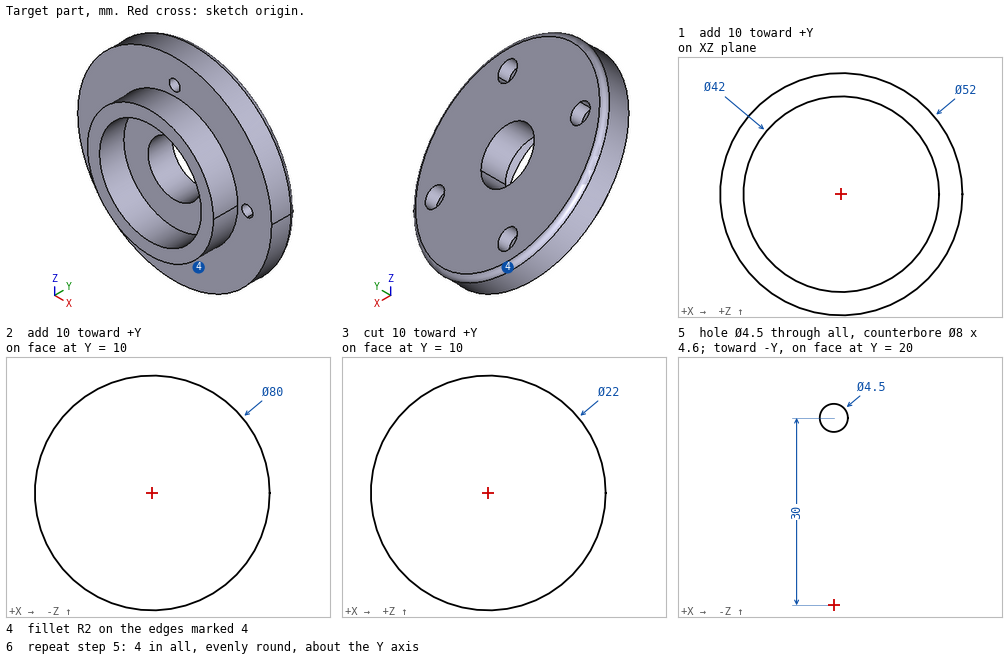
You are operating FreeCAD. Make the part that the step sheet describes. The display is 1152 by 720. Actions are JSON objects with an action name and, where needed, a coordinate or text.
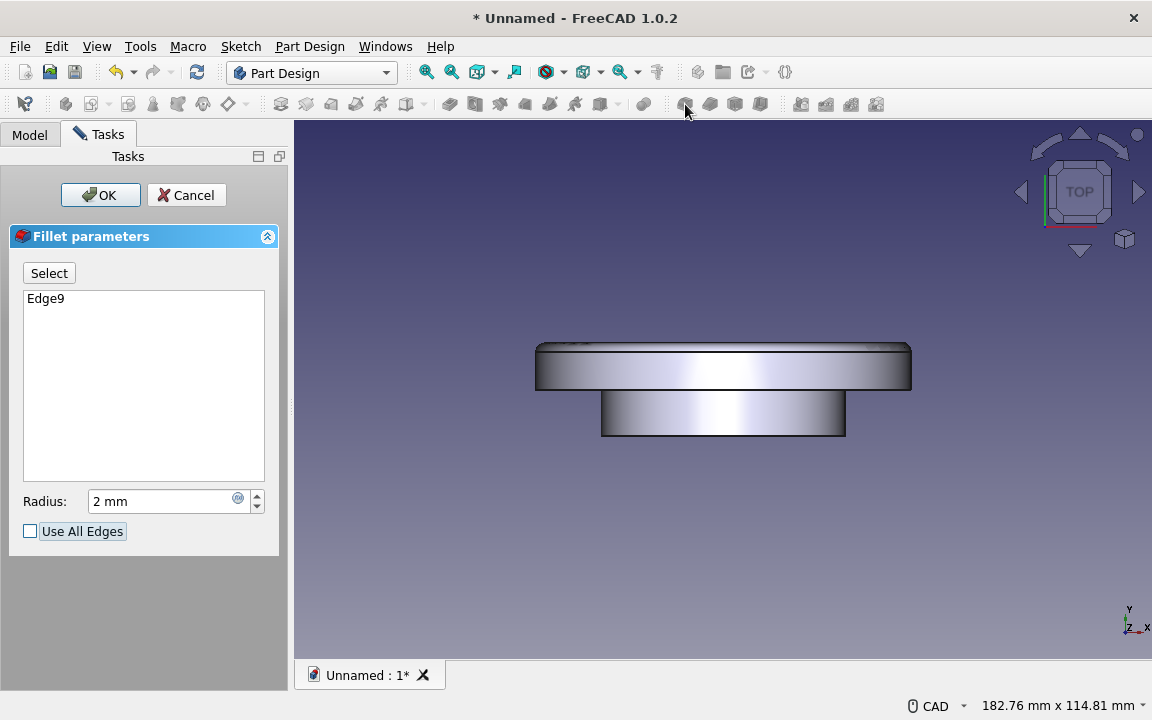
{"action": "left_click", "coordinate": [101, 195]}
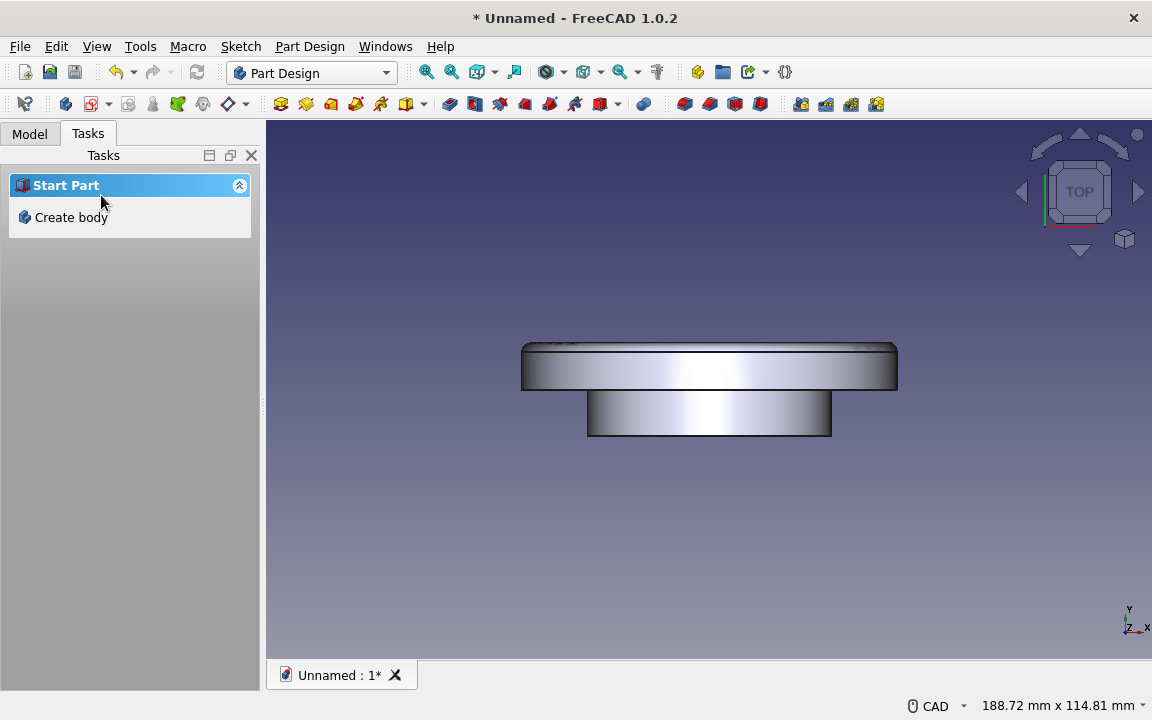
{"action": "key", "text": "v f"}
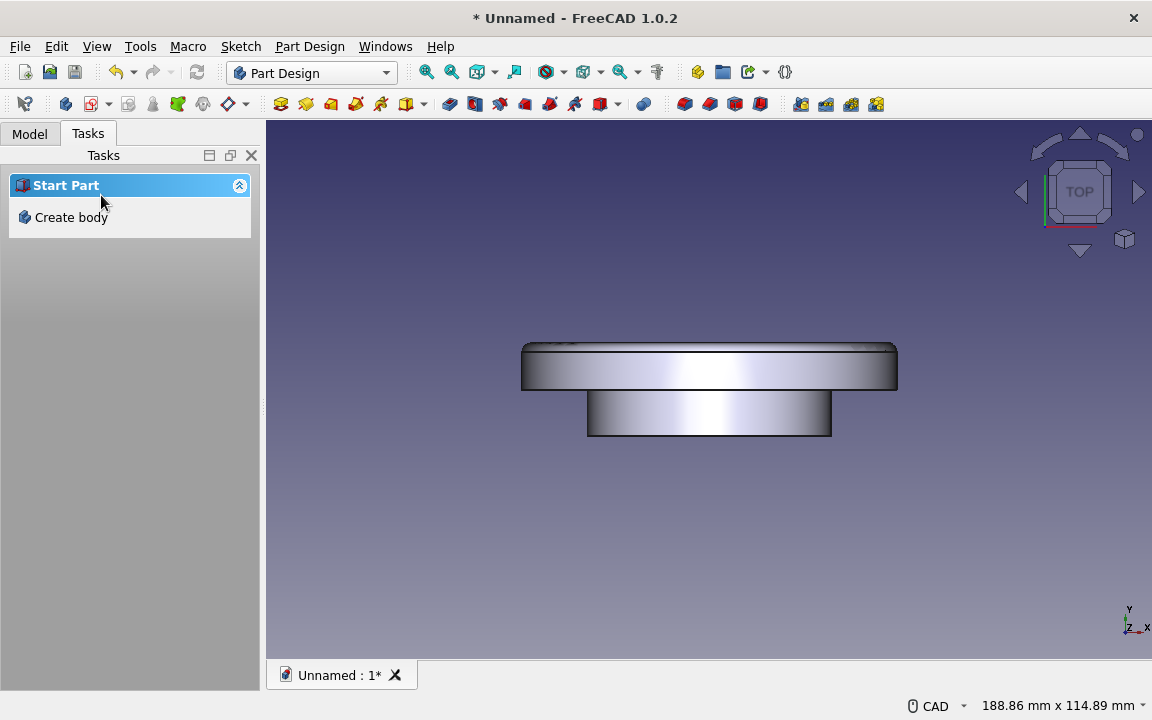
{"action": "key", "text": "4"}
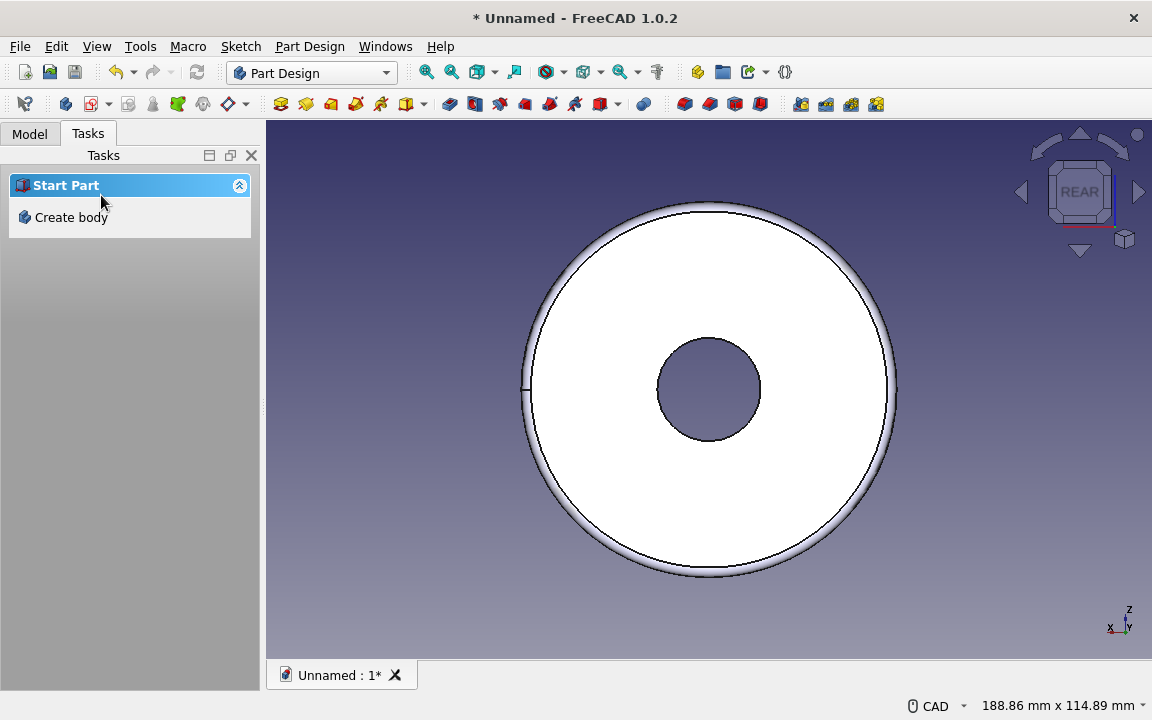
{"action": "left_click", "coordinate": [811, 338]}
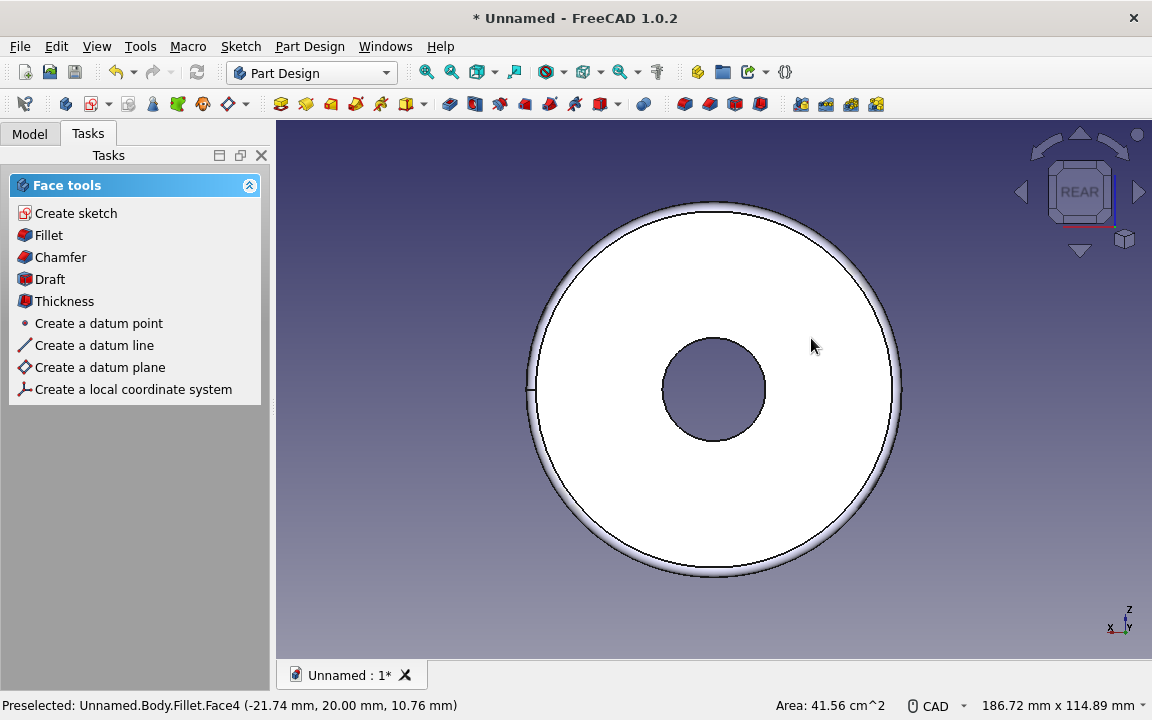
{"action": "left_click", "coordinate": [90, 104]}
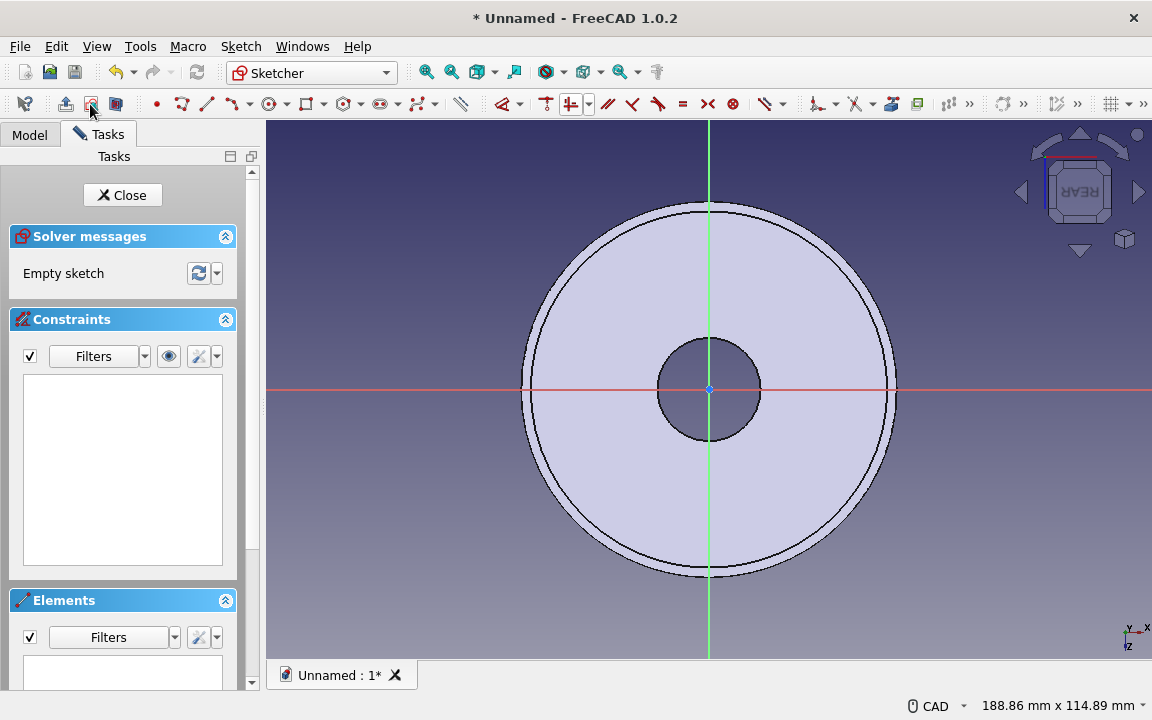
{"action": "scroll", "coordinate": [713, 240], "scroll_direction": "up", "scroll_amount": 14}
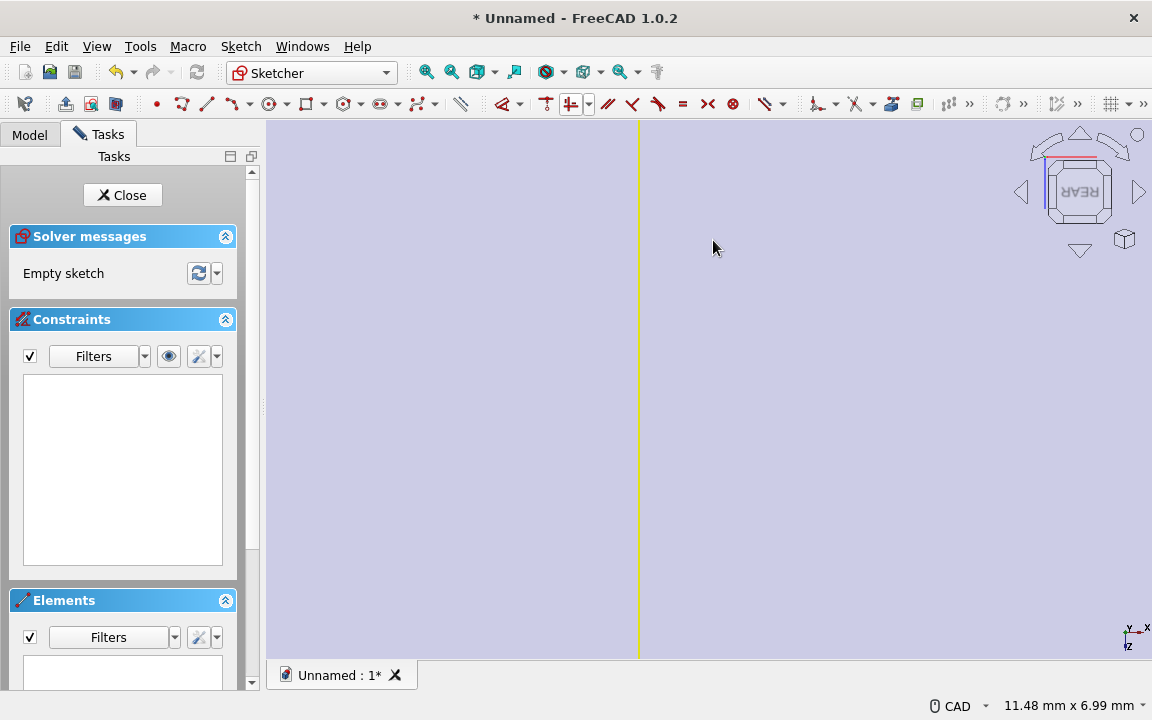
{"action": "left_click", "coordinate": [268, 104]}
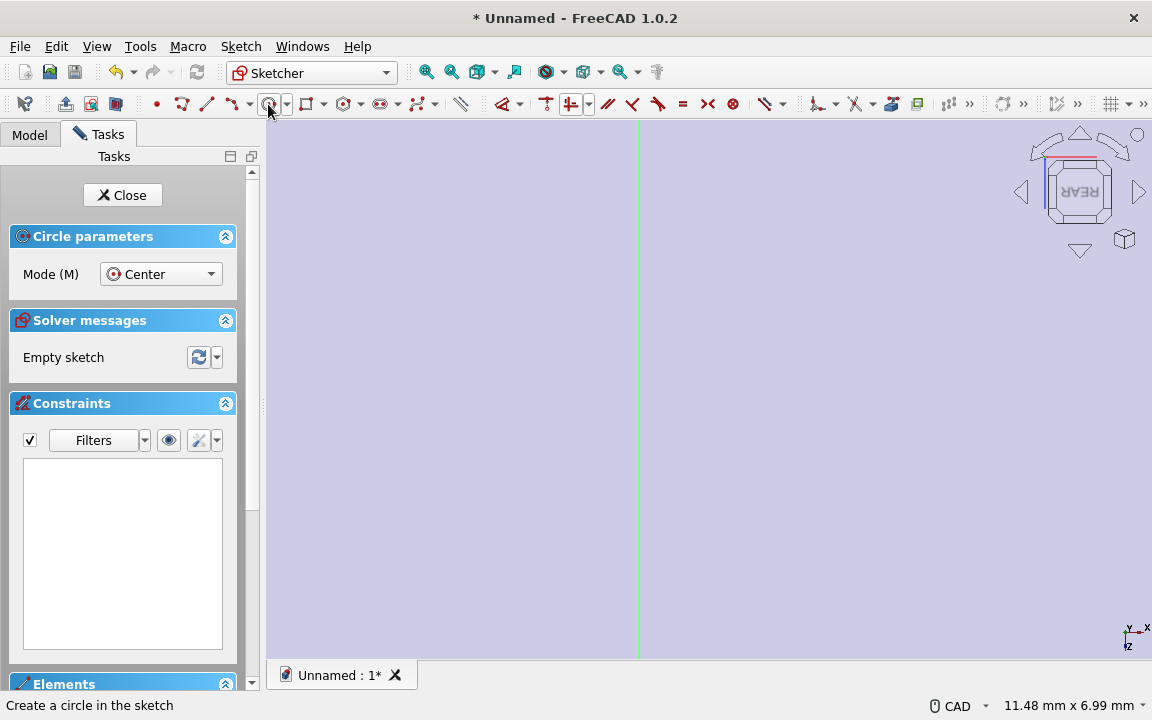
{"action": "left_click", "coordinate": [639, 381]}
{"action": "left_click", "coordinate": [762, 258]}
{"action": "key", "text": "Escape"}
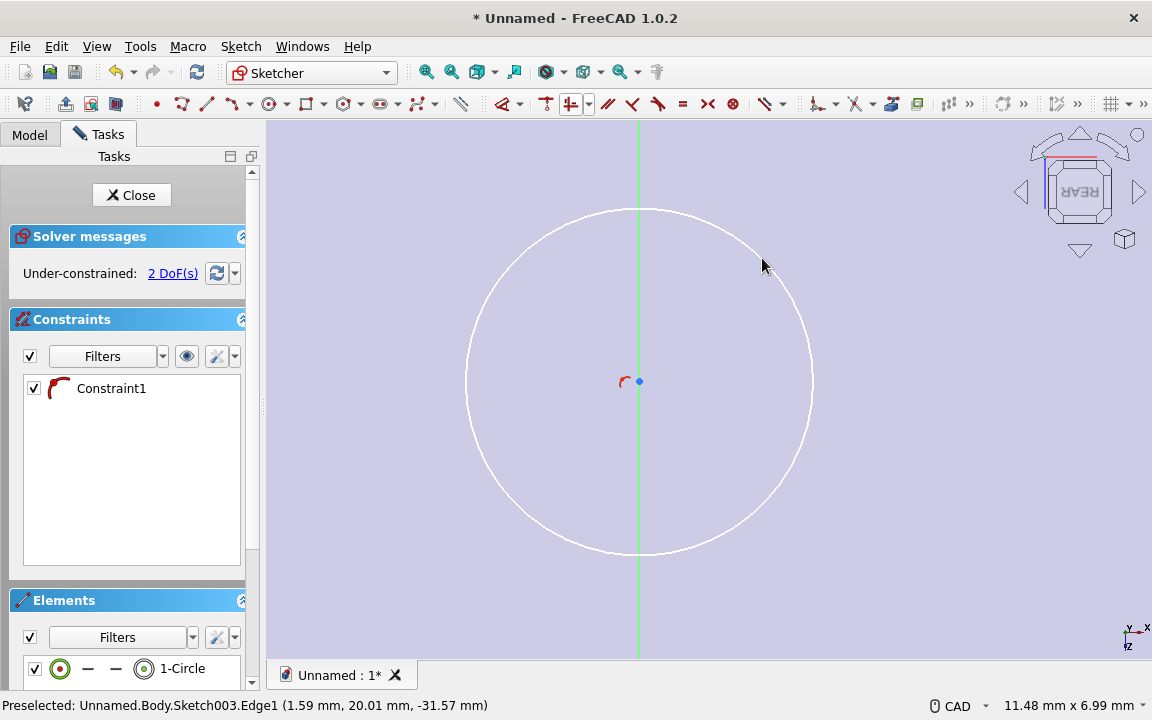
{"action": "key", "text": "d"}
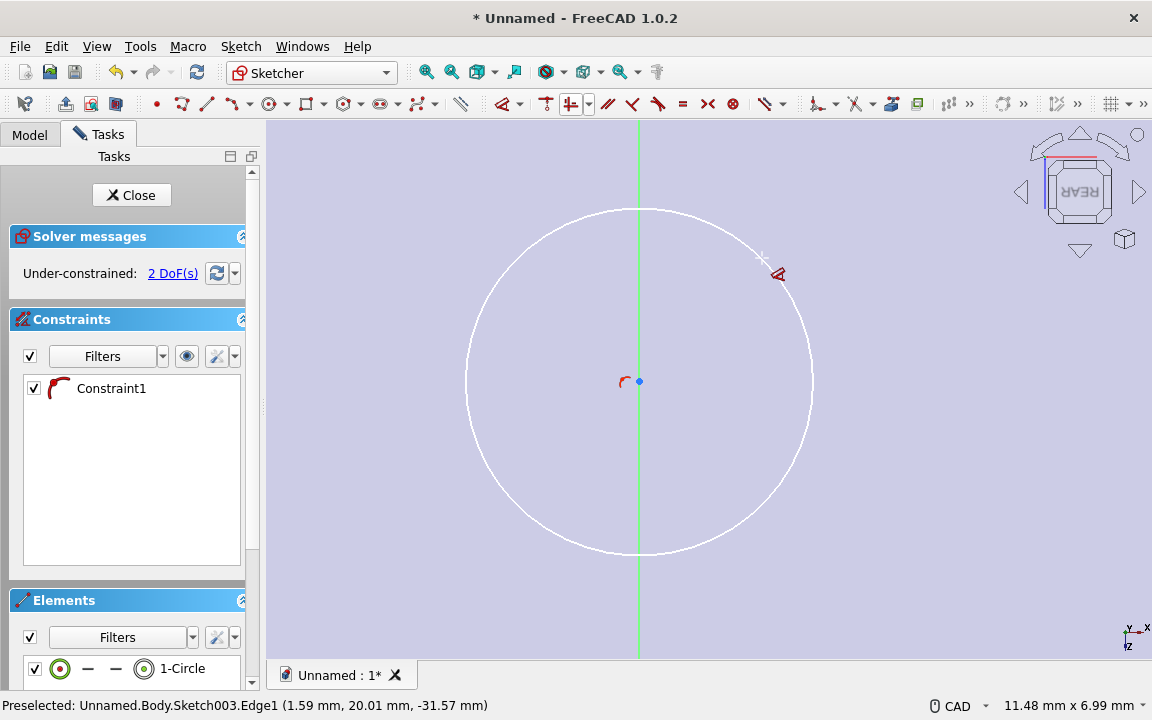
{"action": "left_click", "coordinate": [762, 259]}
{"action": "left_click", "coordinate": [785, 236]}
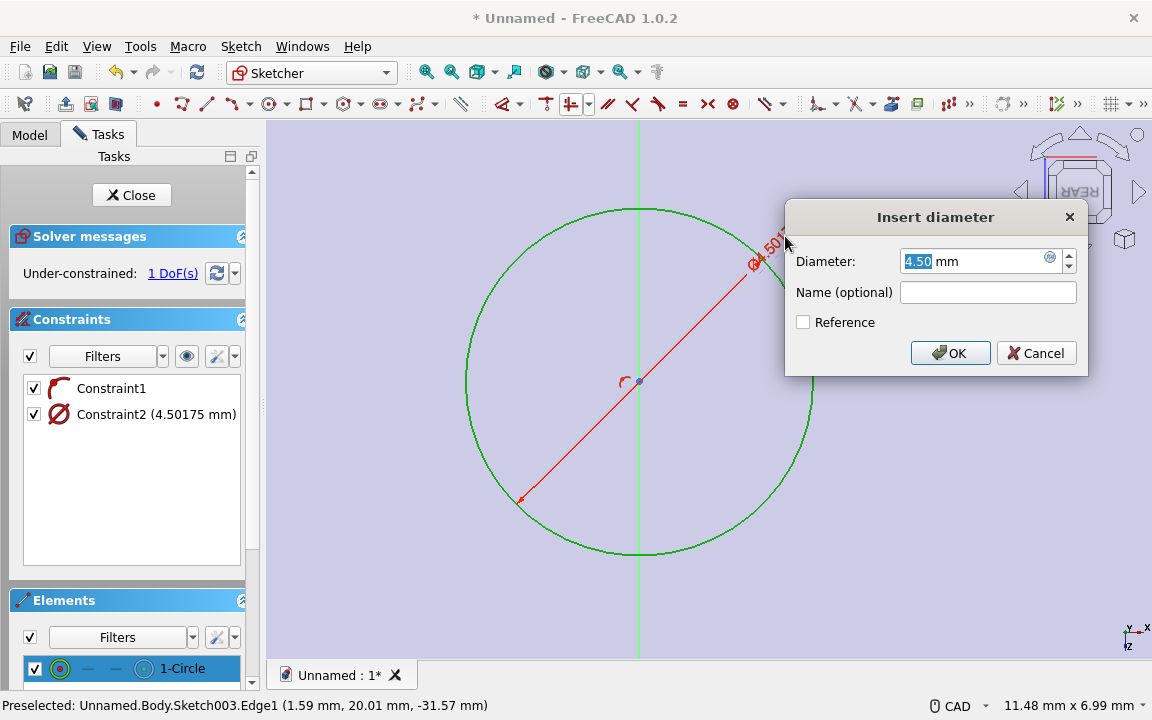
{"action": "type", "text": "4.5"}
{"action": "key", "text": "Return"}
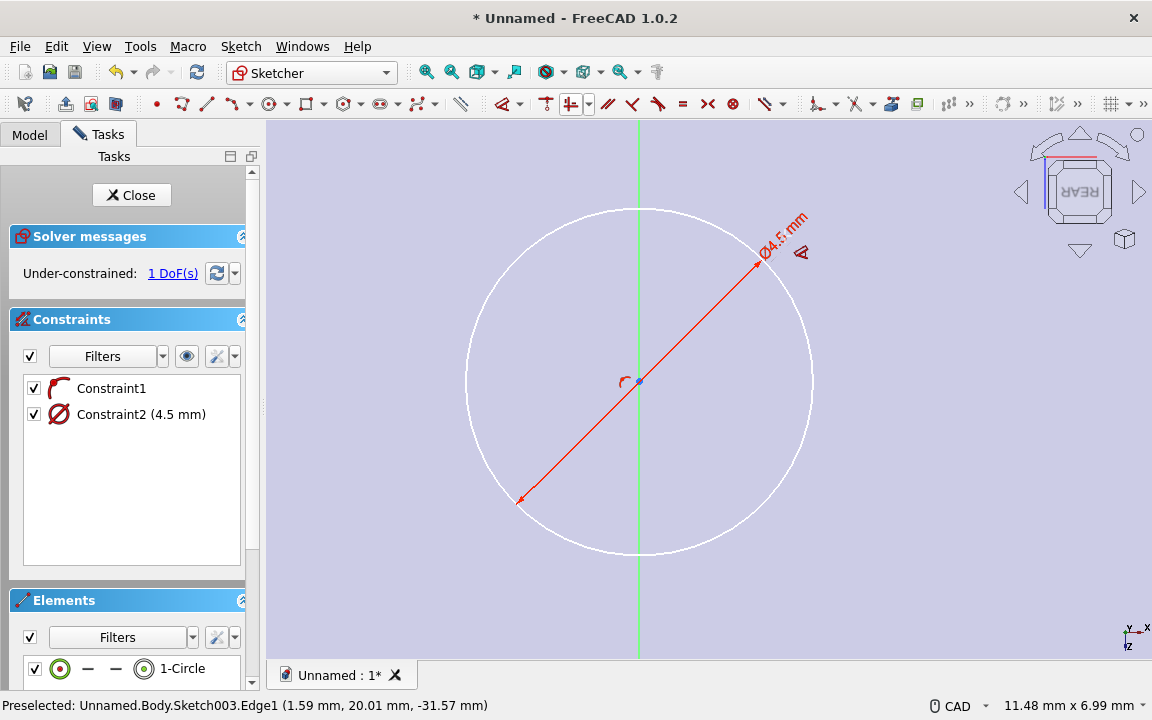
{"action": "left_click", "coordinate": [639, 382]}
{"action": "left_click", "coordinate": [673, 507]}